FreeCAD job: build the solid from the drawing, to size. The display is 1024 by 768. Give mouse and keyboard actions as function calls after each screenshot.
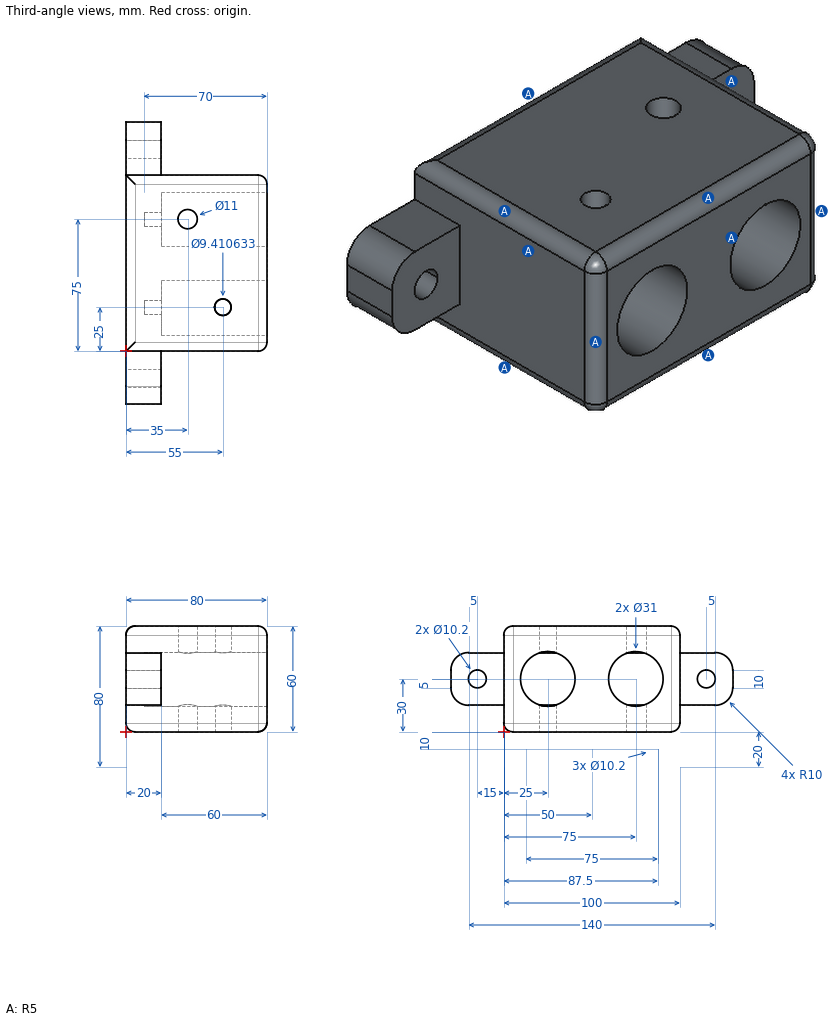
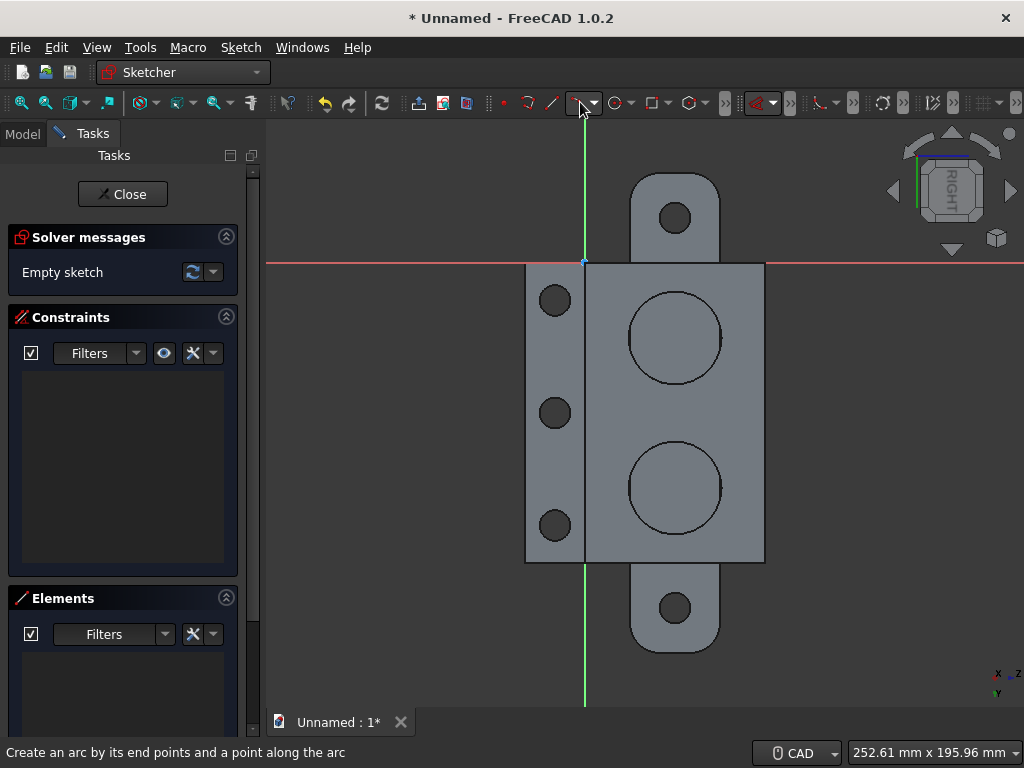
key(q)
key(s)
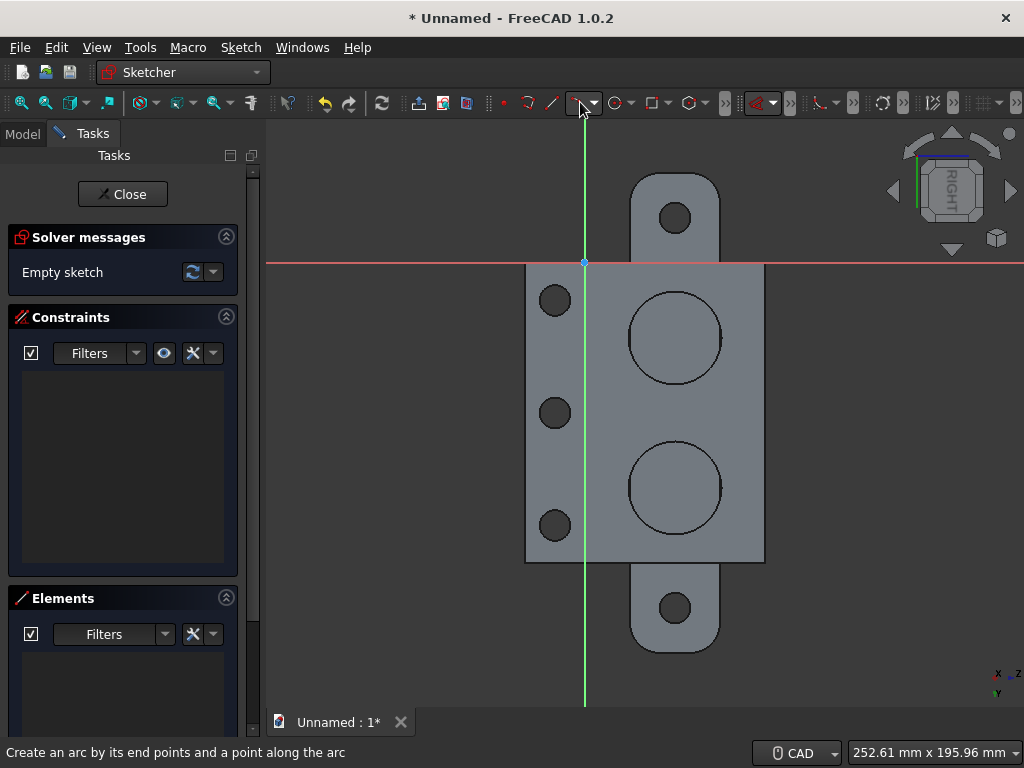
click(652, 104)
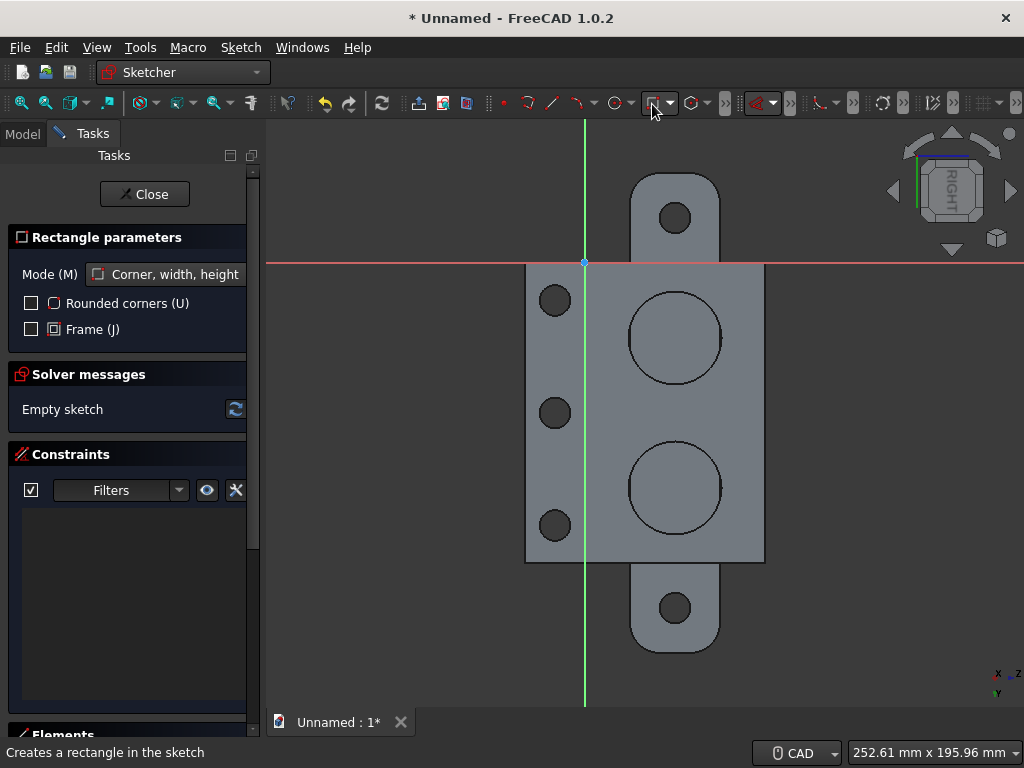
click(585, 263)
move(525, 563)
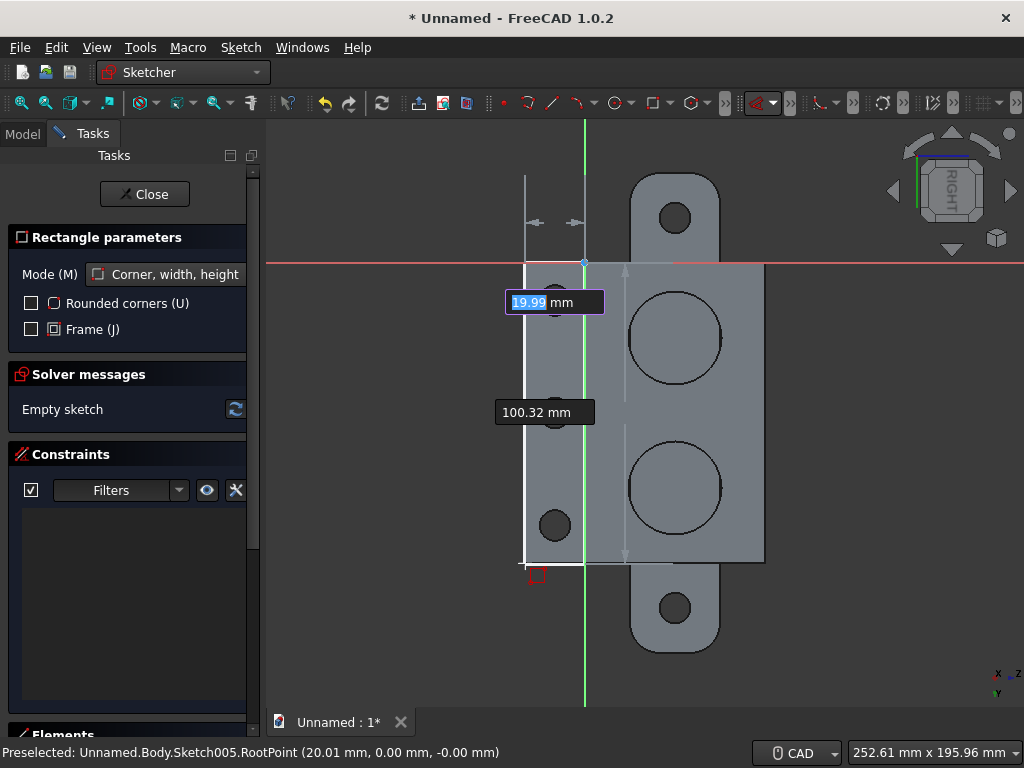
text(20)
key(Tab)
text(100)
key(Return)
key(Escape)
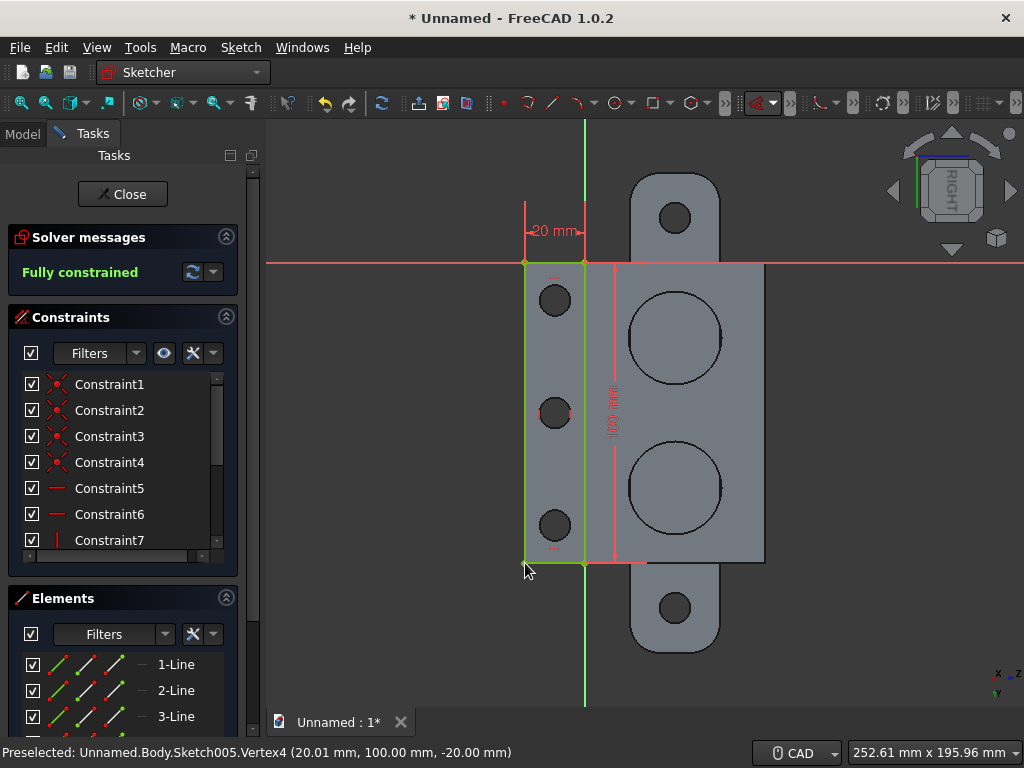
click(123, 194)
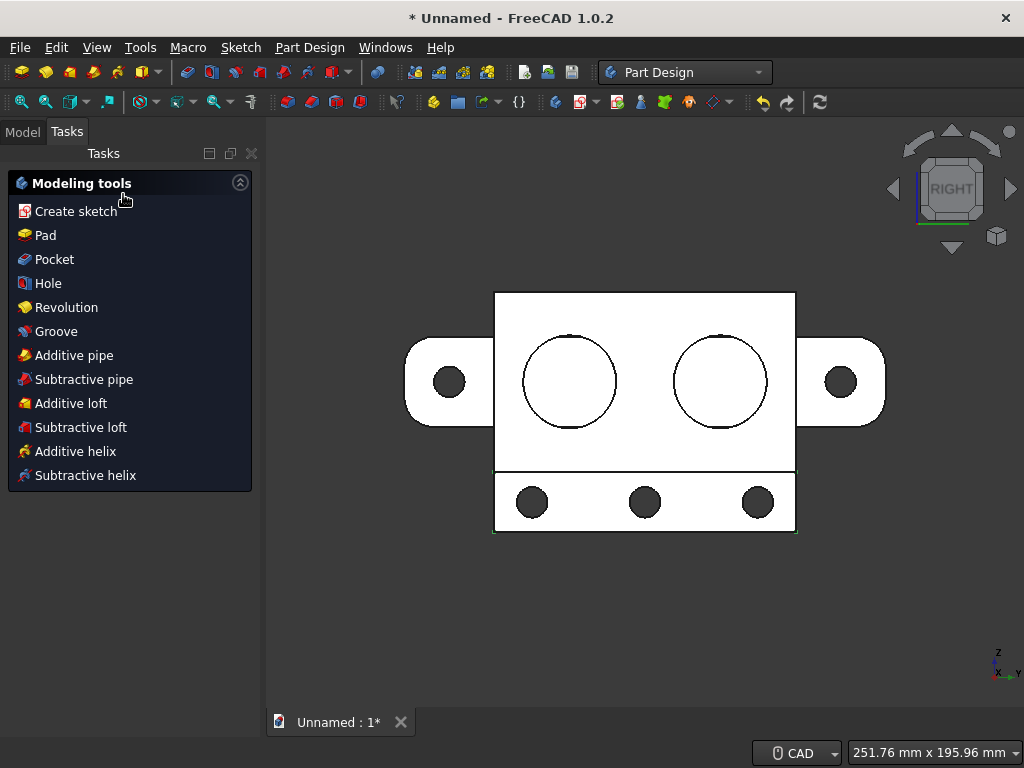
click(188, 72)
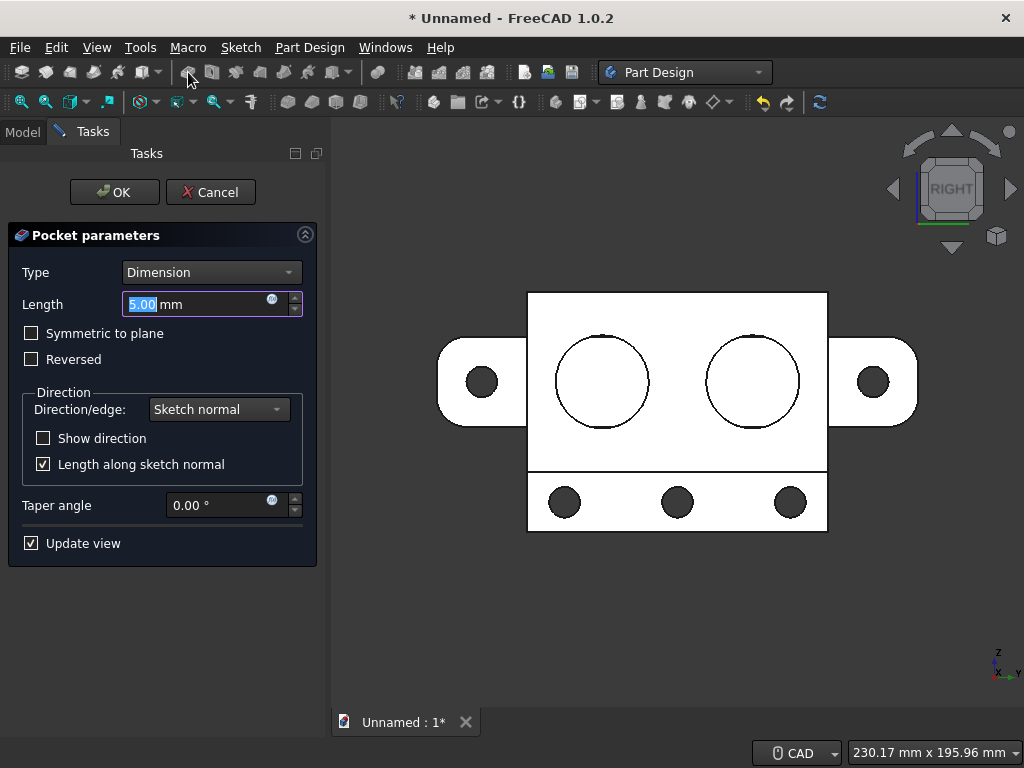
text(20)
key(Tab)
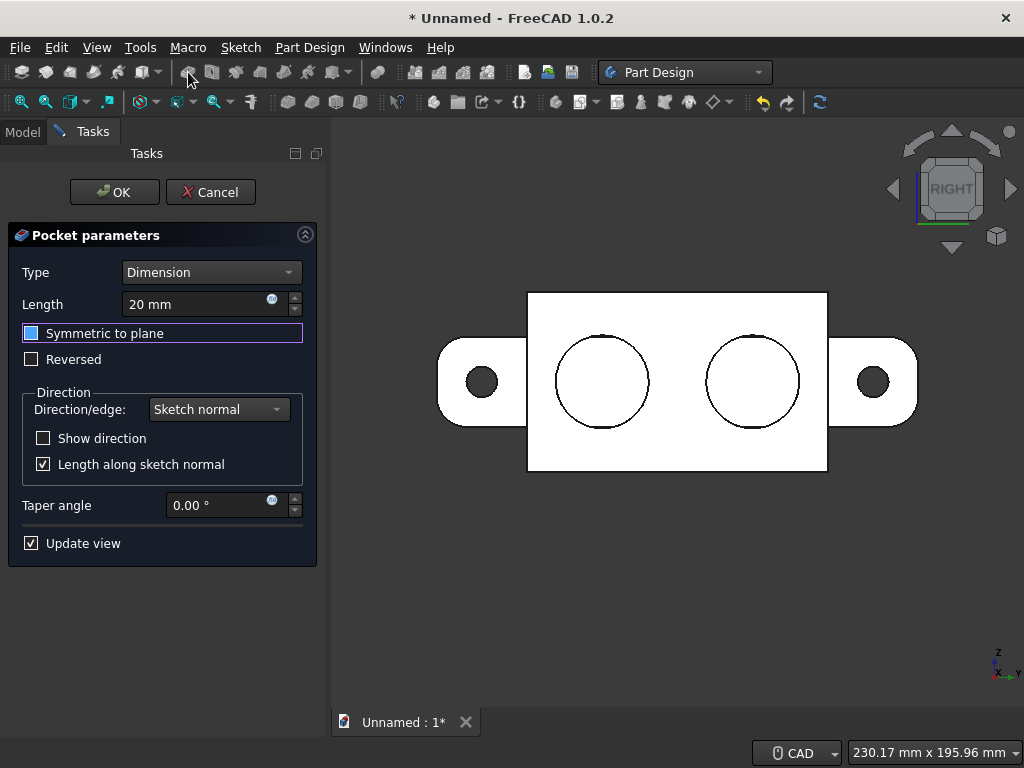
click(115, 192)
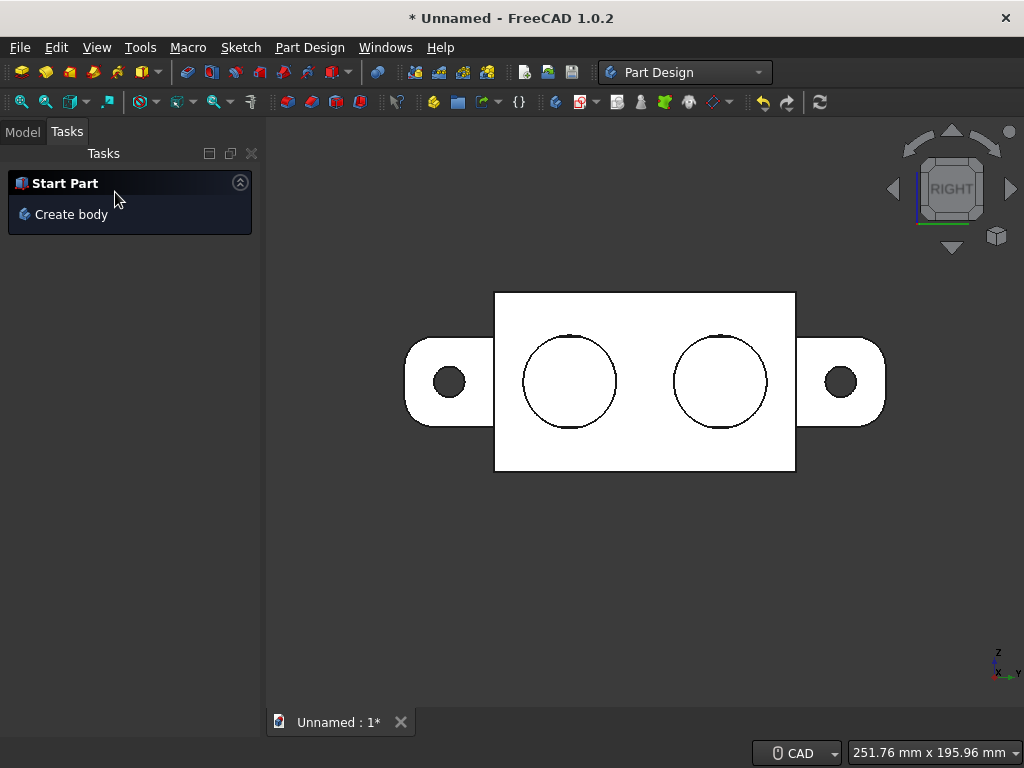
click(796, 381)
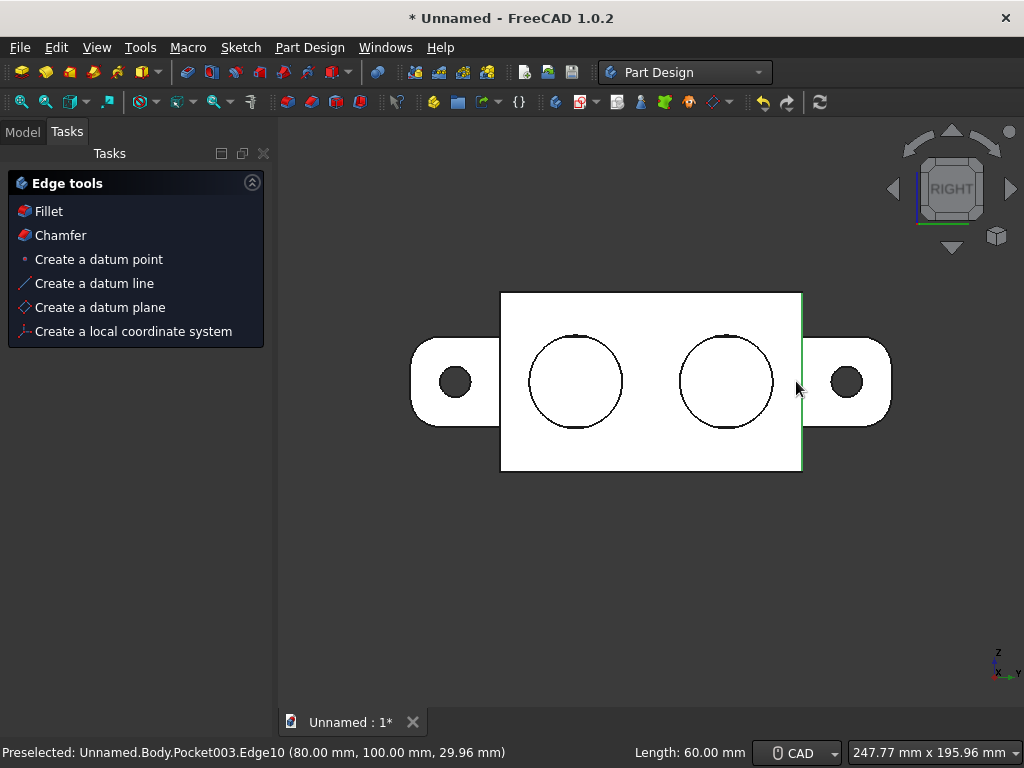
click(651, 471, ctrl)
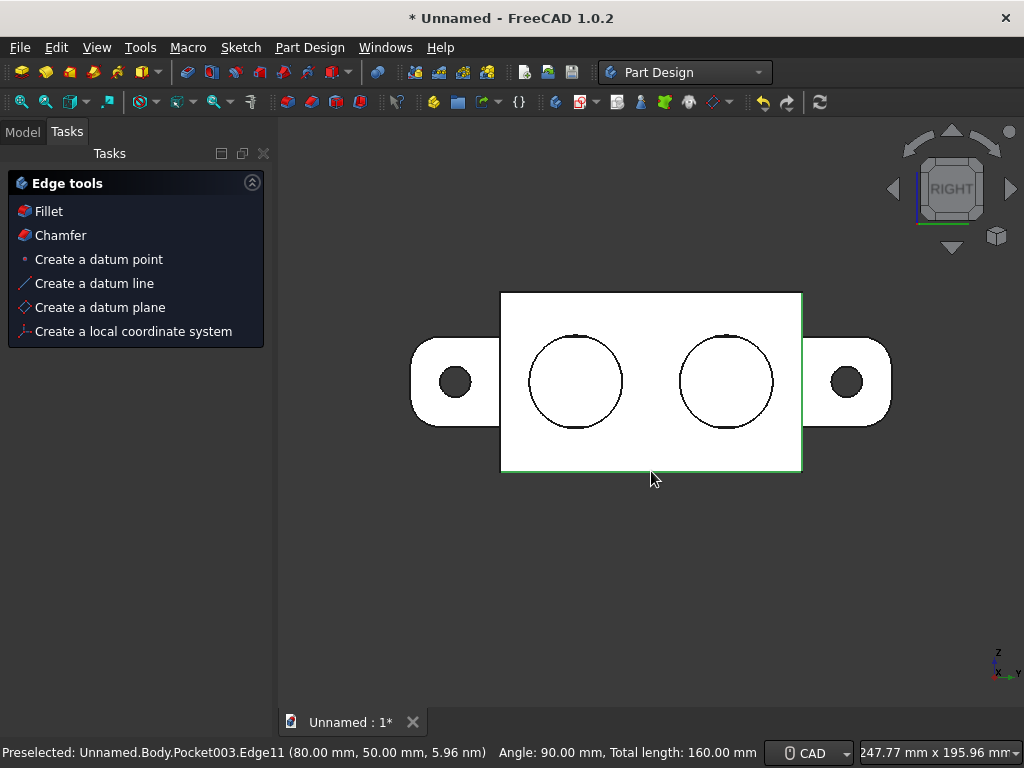
key(0)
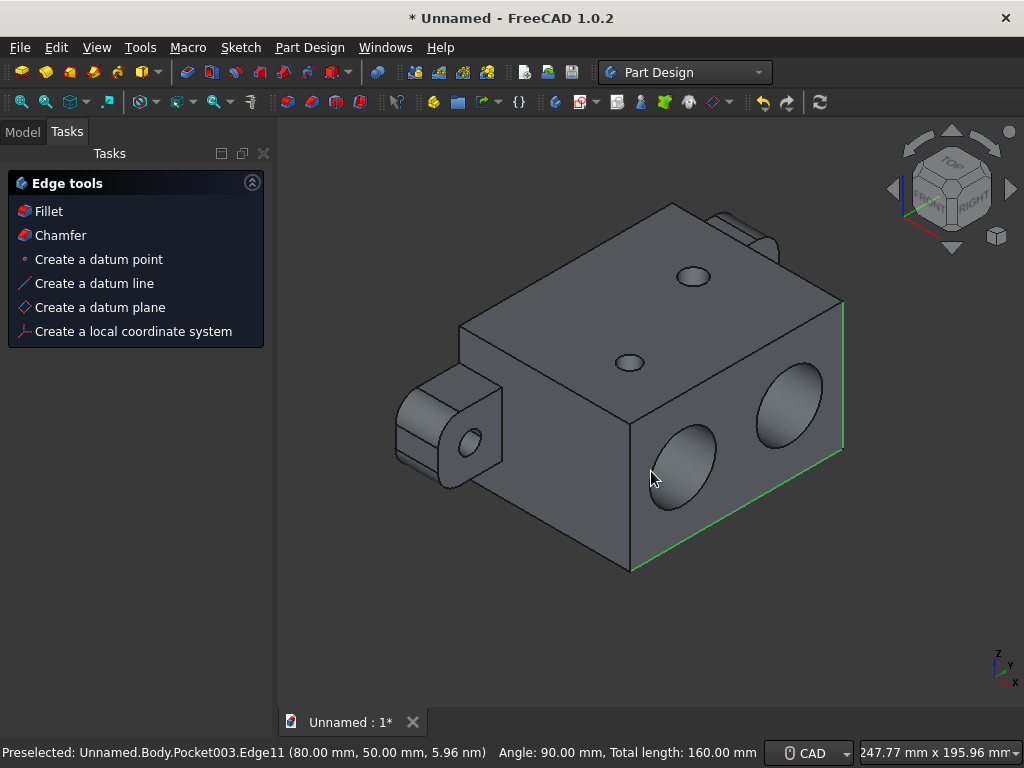
click(736, 362, ctrl)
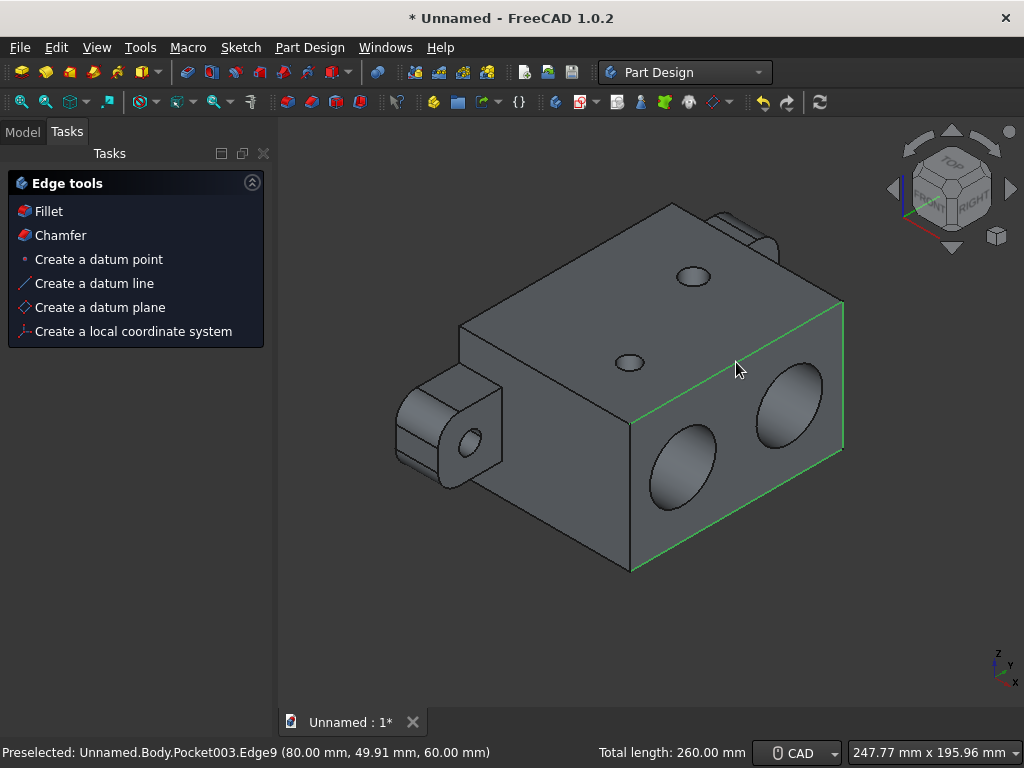
click(630, 497, ctrl)